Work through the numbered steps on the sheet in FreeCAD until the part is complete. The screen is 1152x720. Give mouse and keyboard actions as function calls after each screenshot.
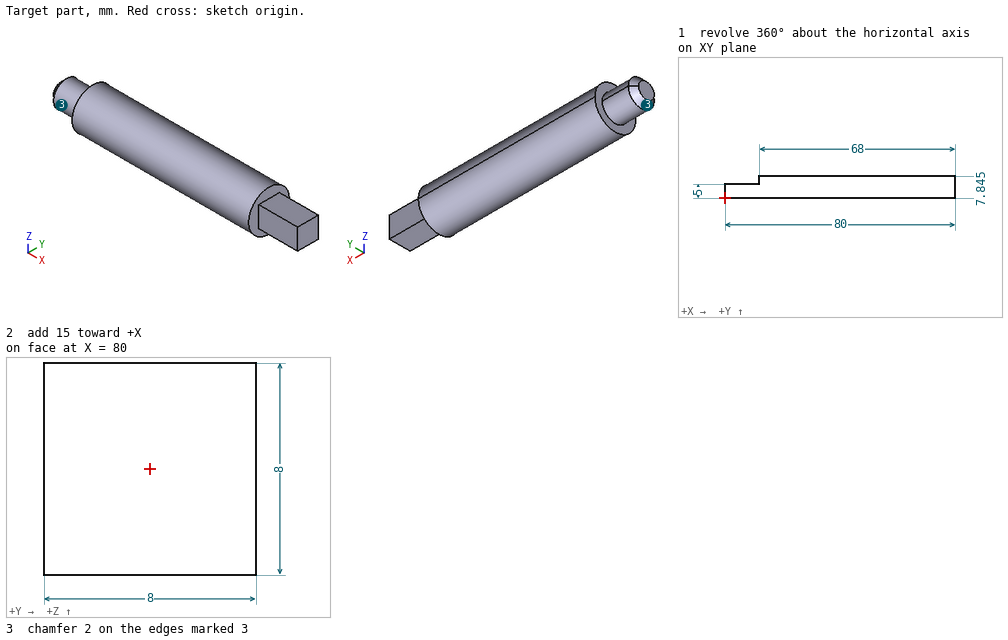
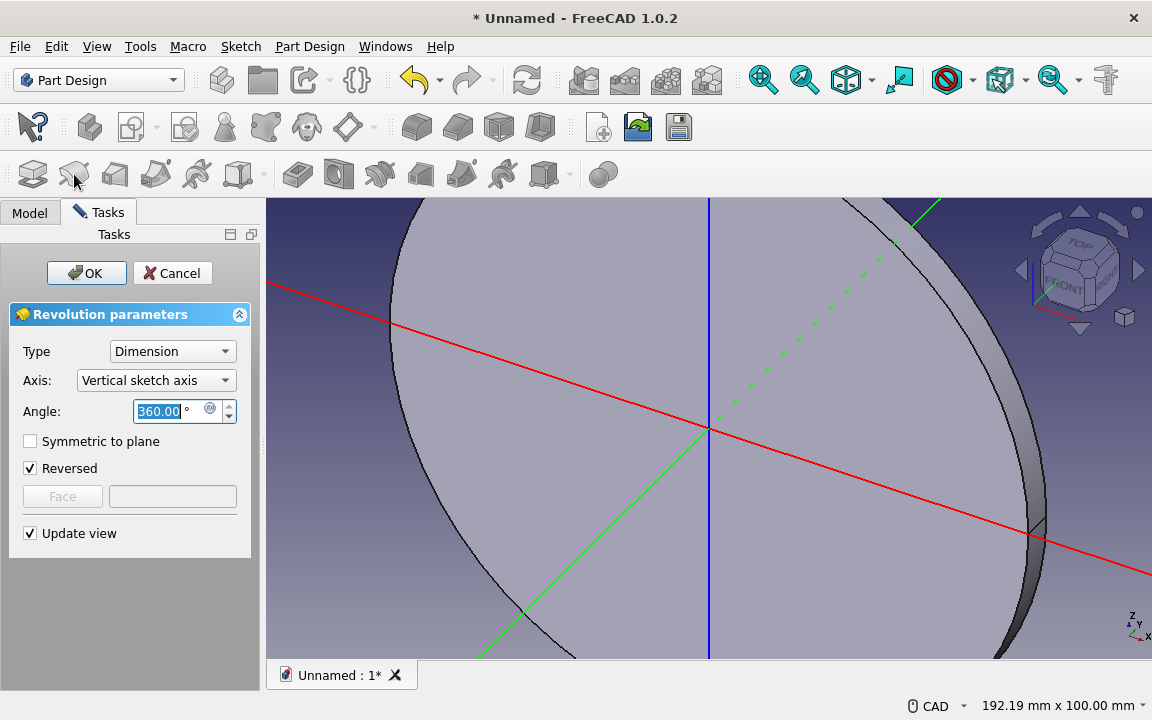
click(157, 380)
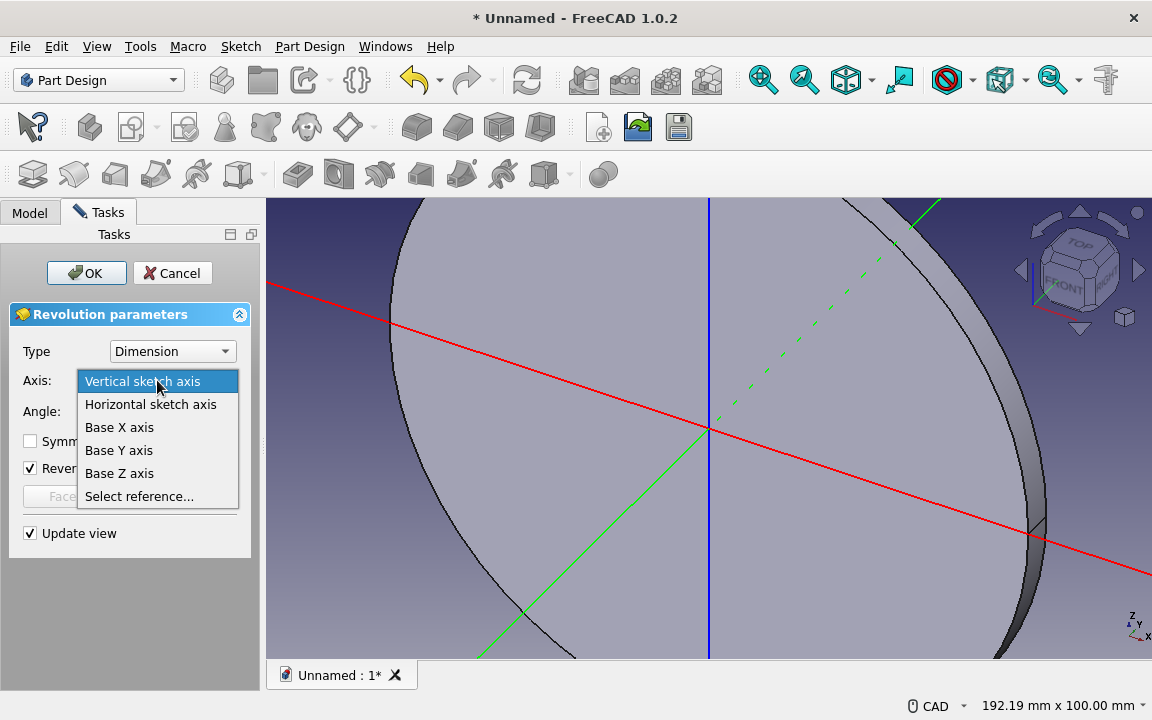
click(156, 404)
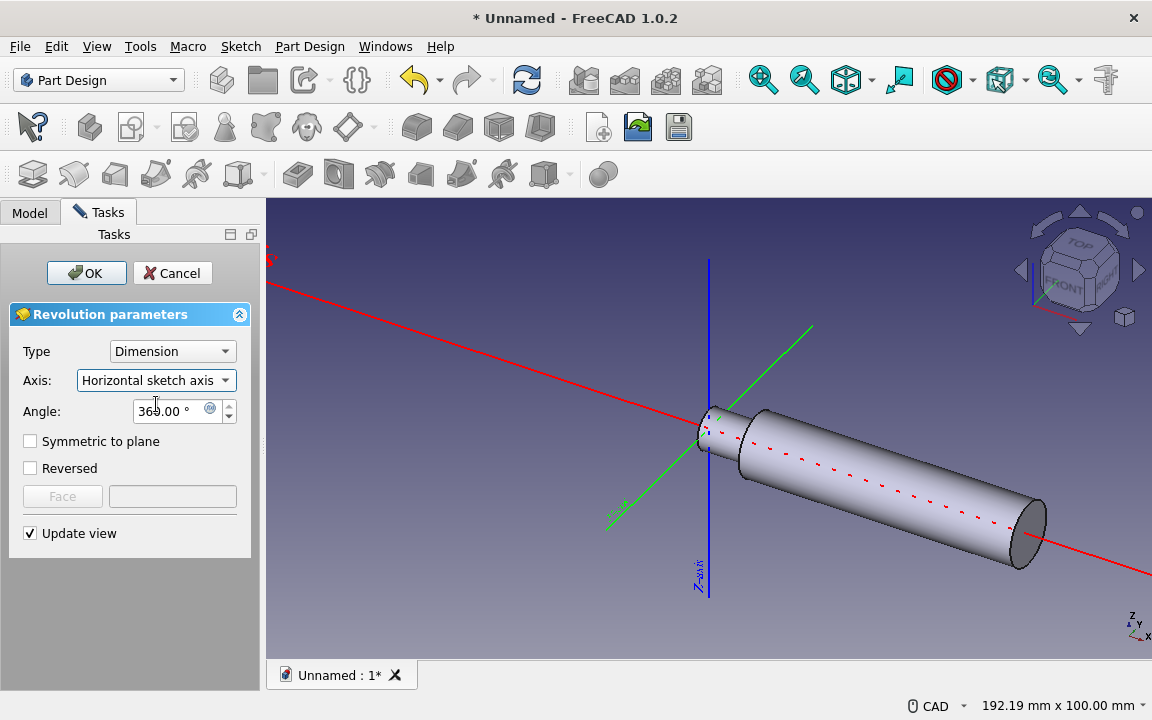
click(87, 273)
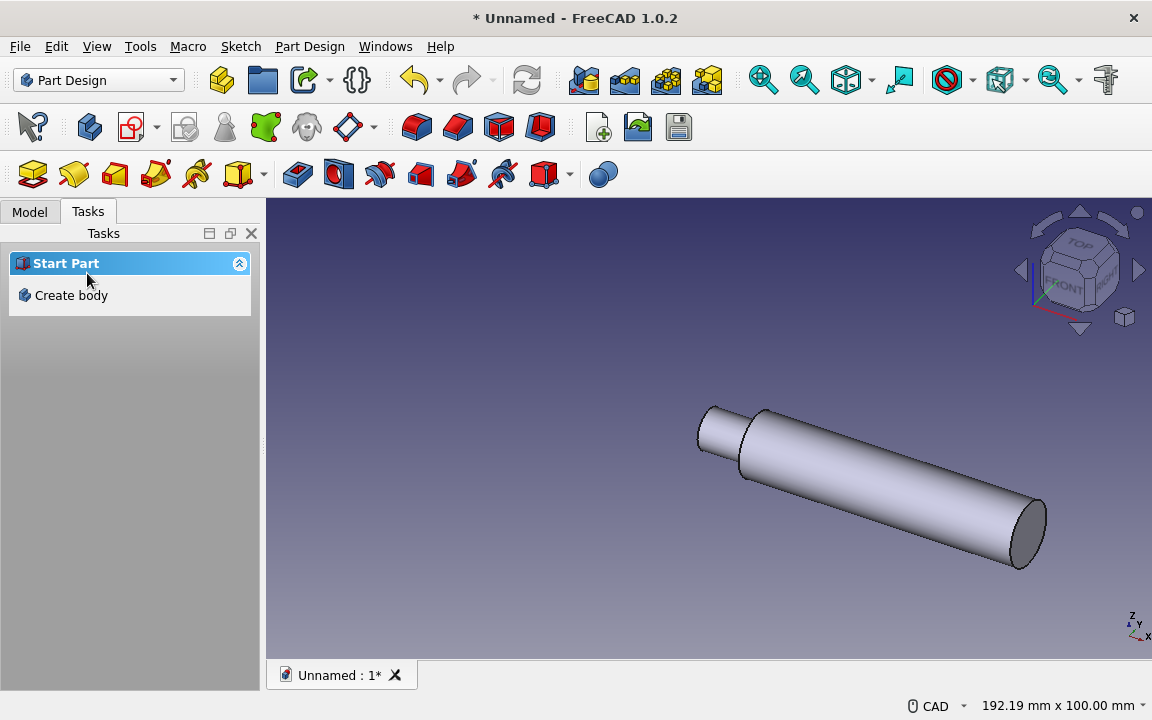
click(764, 80)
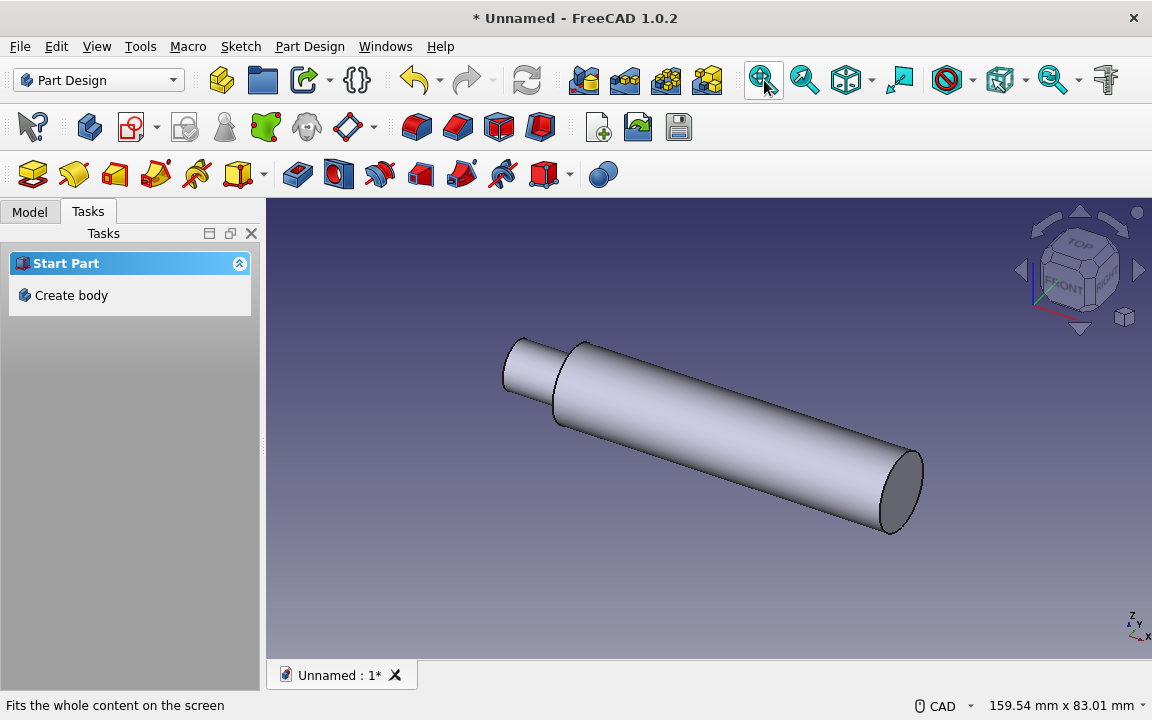
click(901, 491)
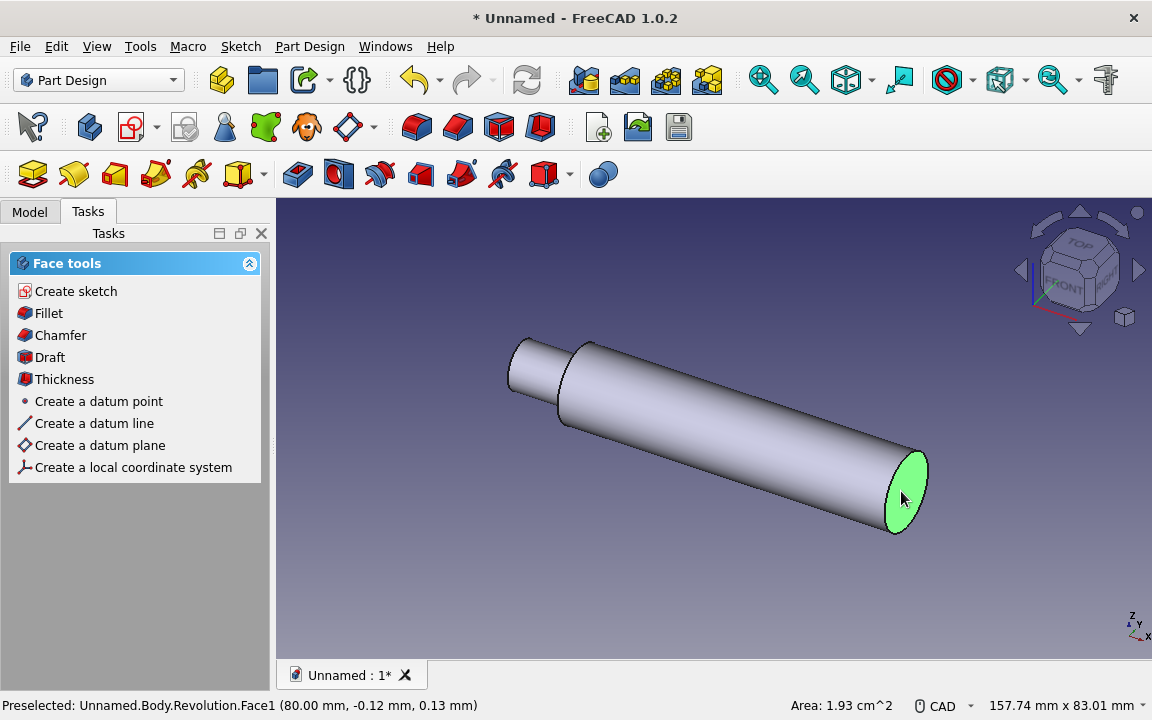
click(130, 128)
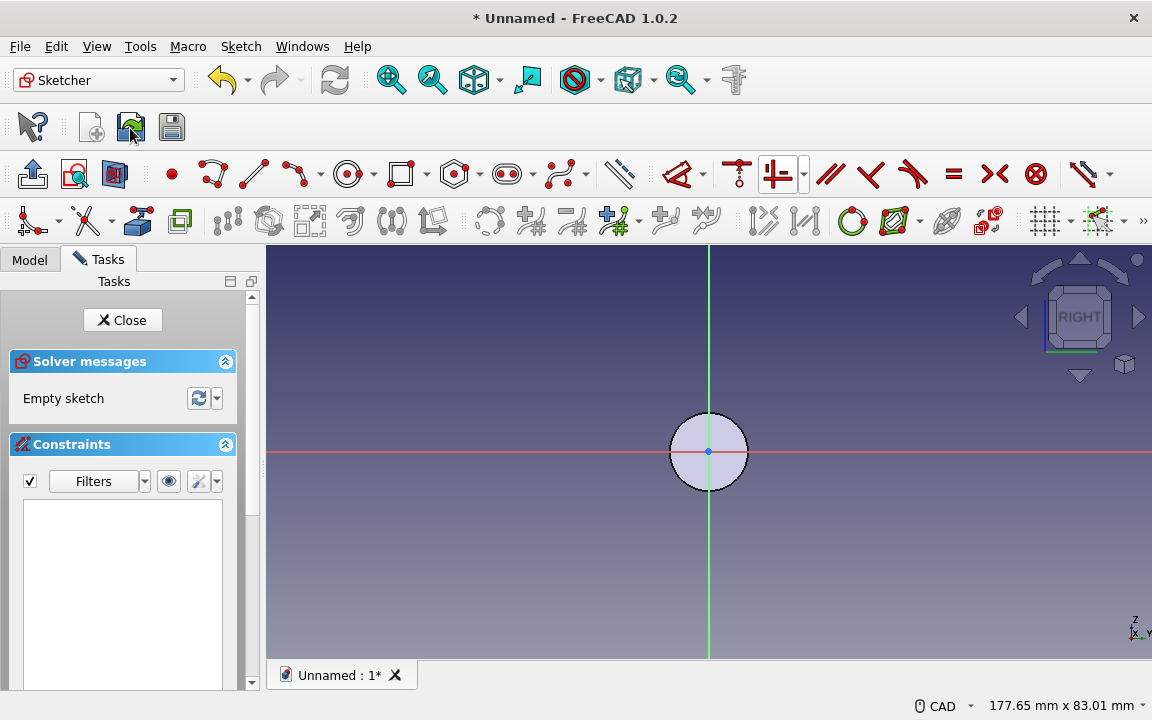
scroll(722, 452, up, 9)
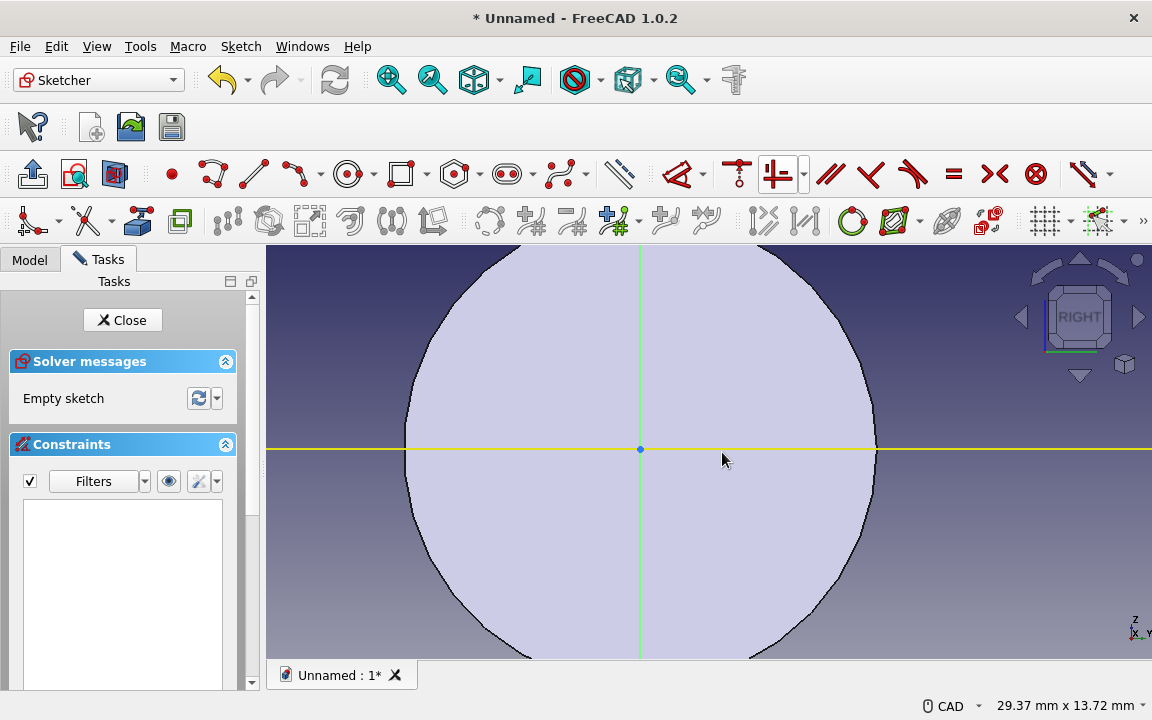
click(426, 174)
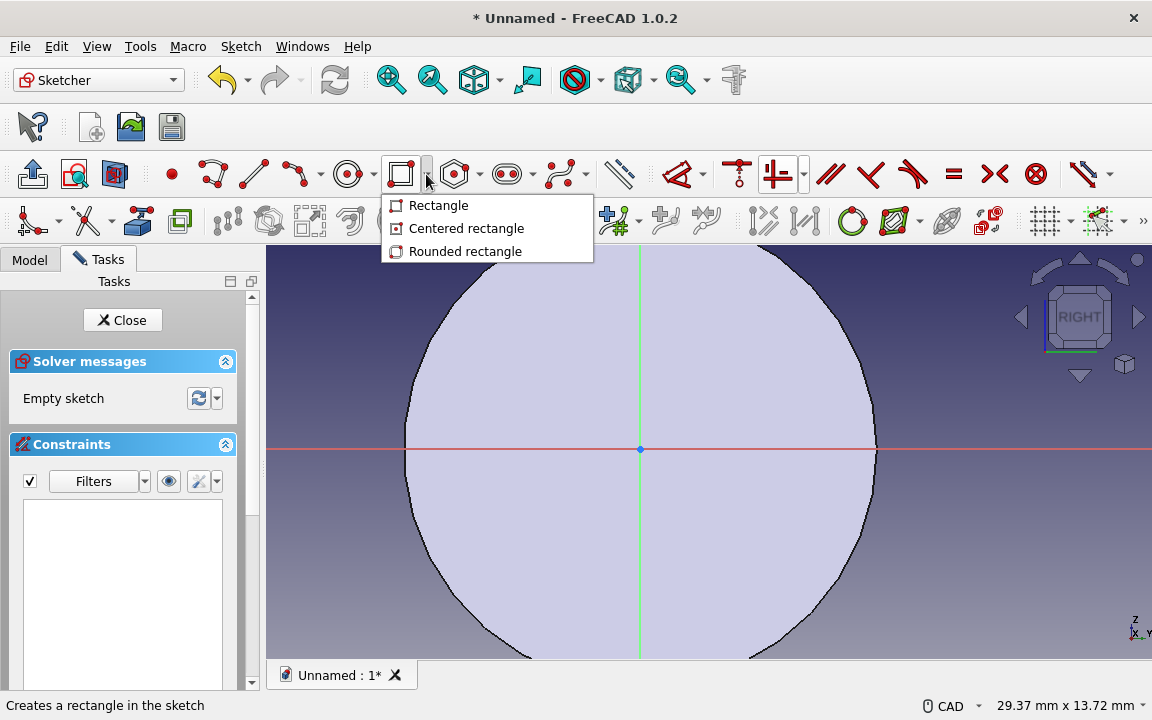
click(488, 228)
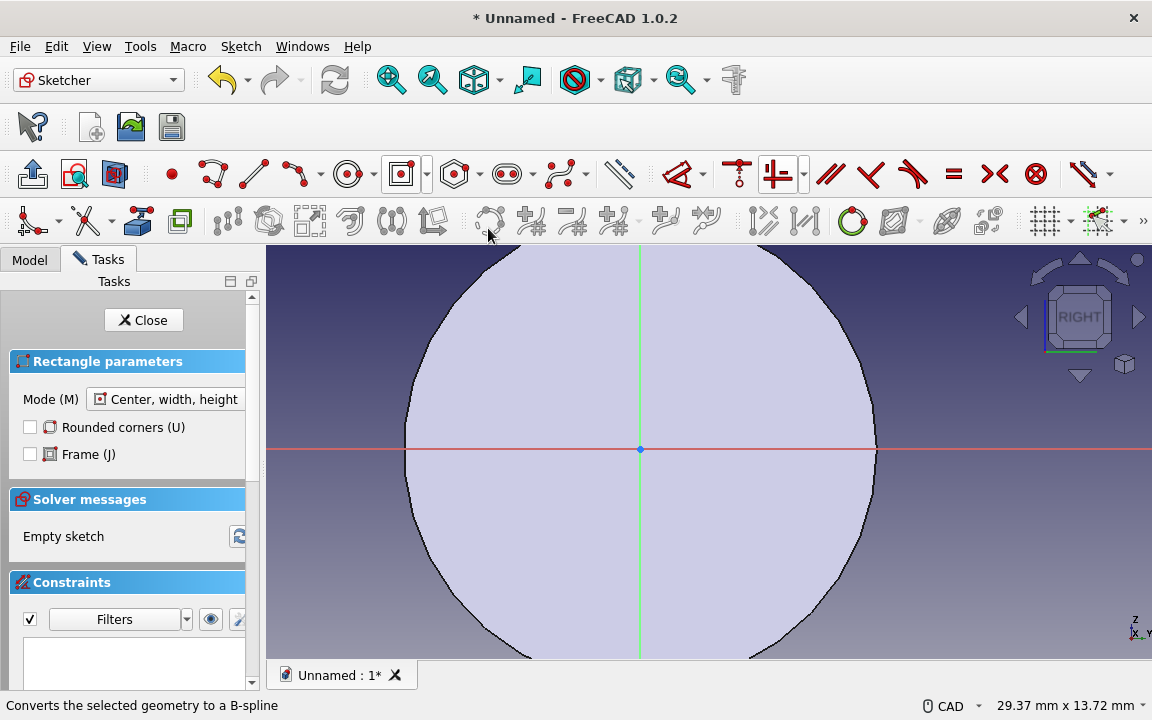
click(640, 449)
click(761, 329)
key(Escape)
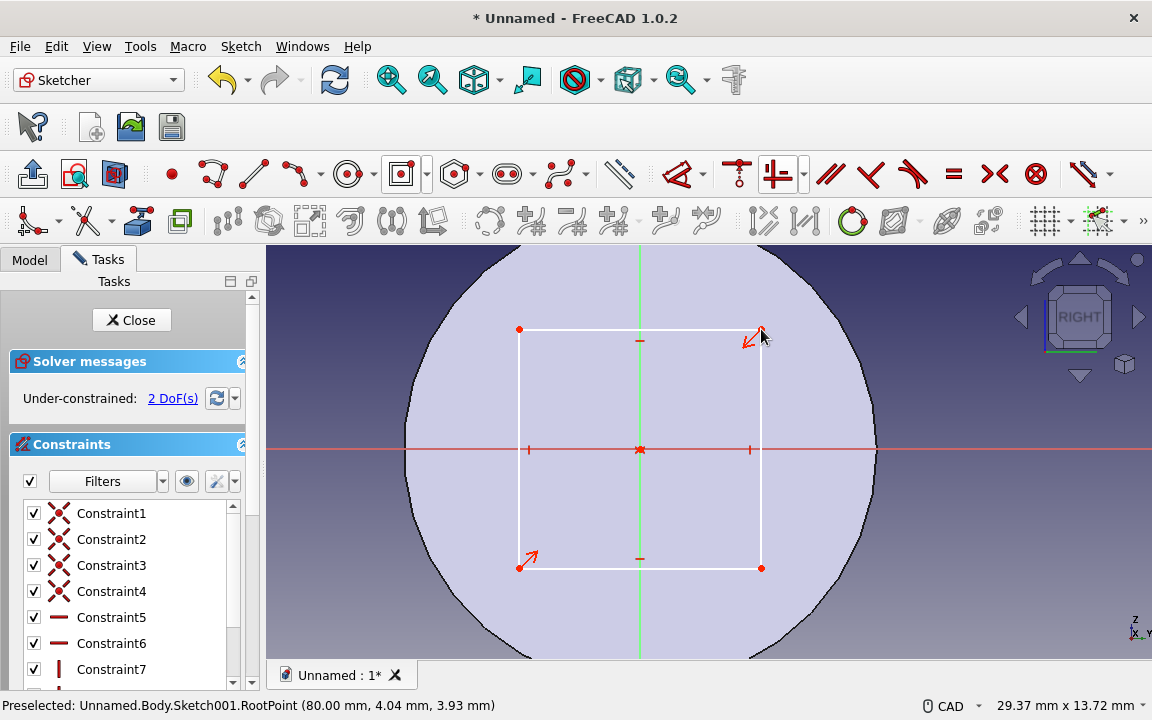
click(676, 174)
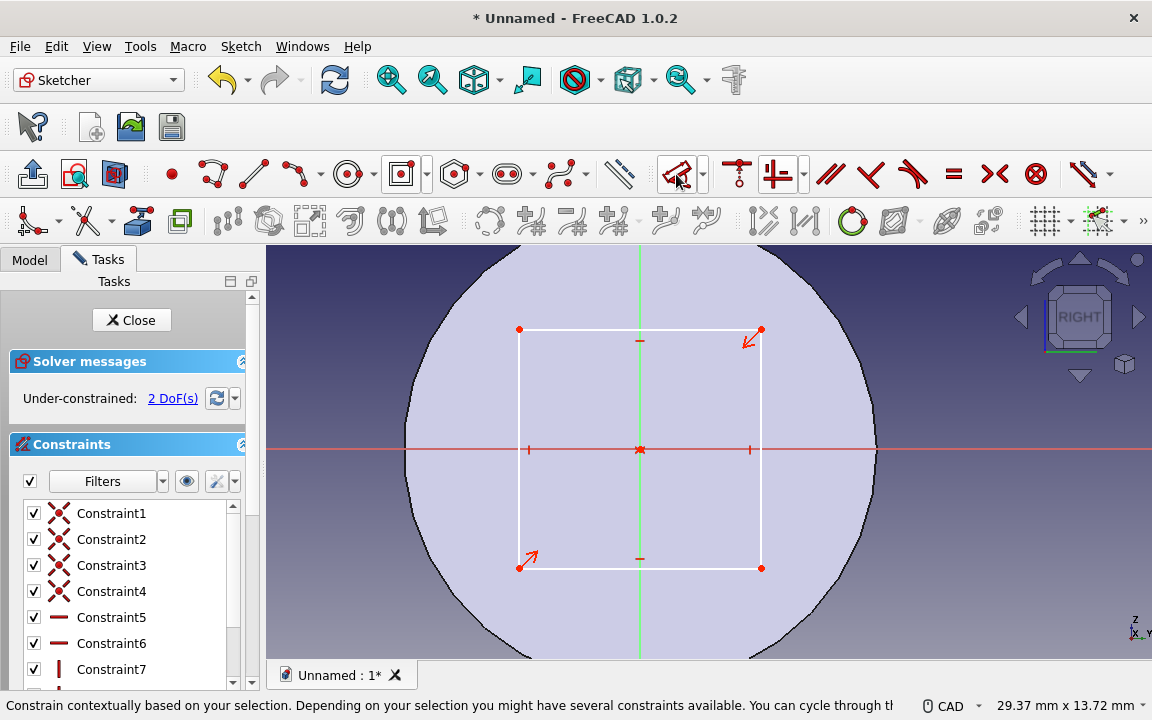
click(592, 569)
click(585, 603)